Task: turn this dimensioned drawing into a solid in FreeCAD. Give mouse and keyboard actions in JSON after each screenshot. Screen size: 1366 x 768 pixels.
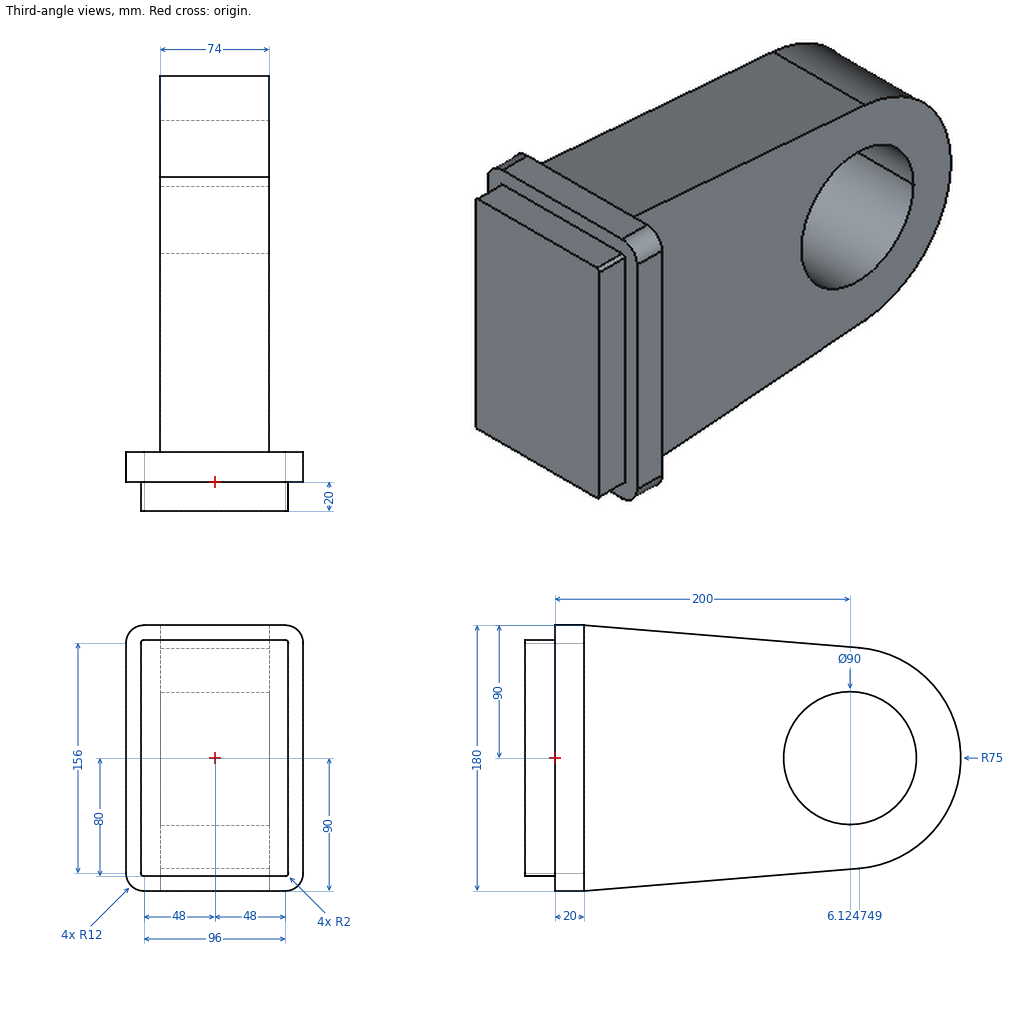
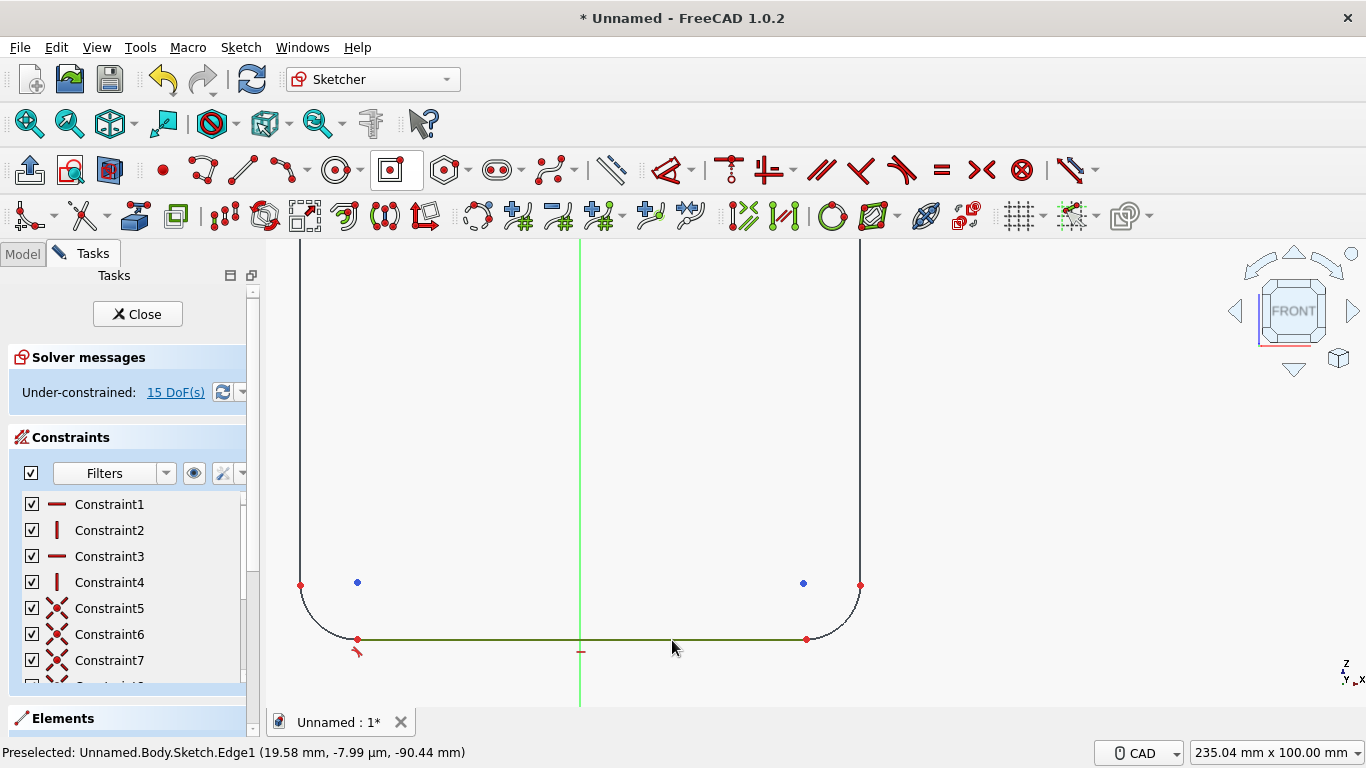
{"action": "left_click", "coordinate": [830, 633]}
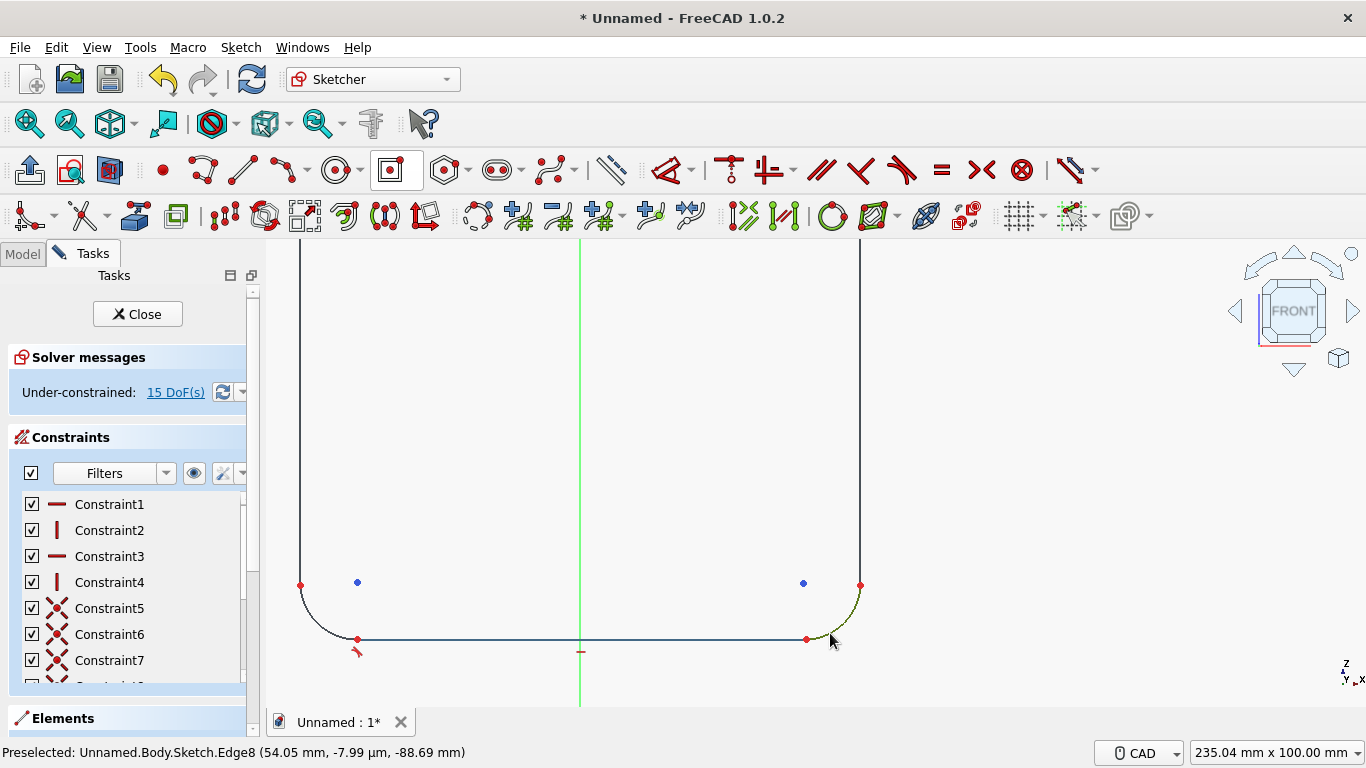
{"action": "left_click", "coordinate": [902, 170]}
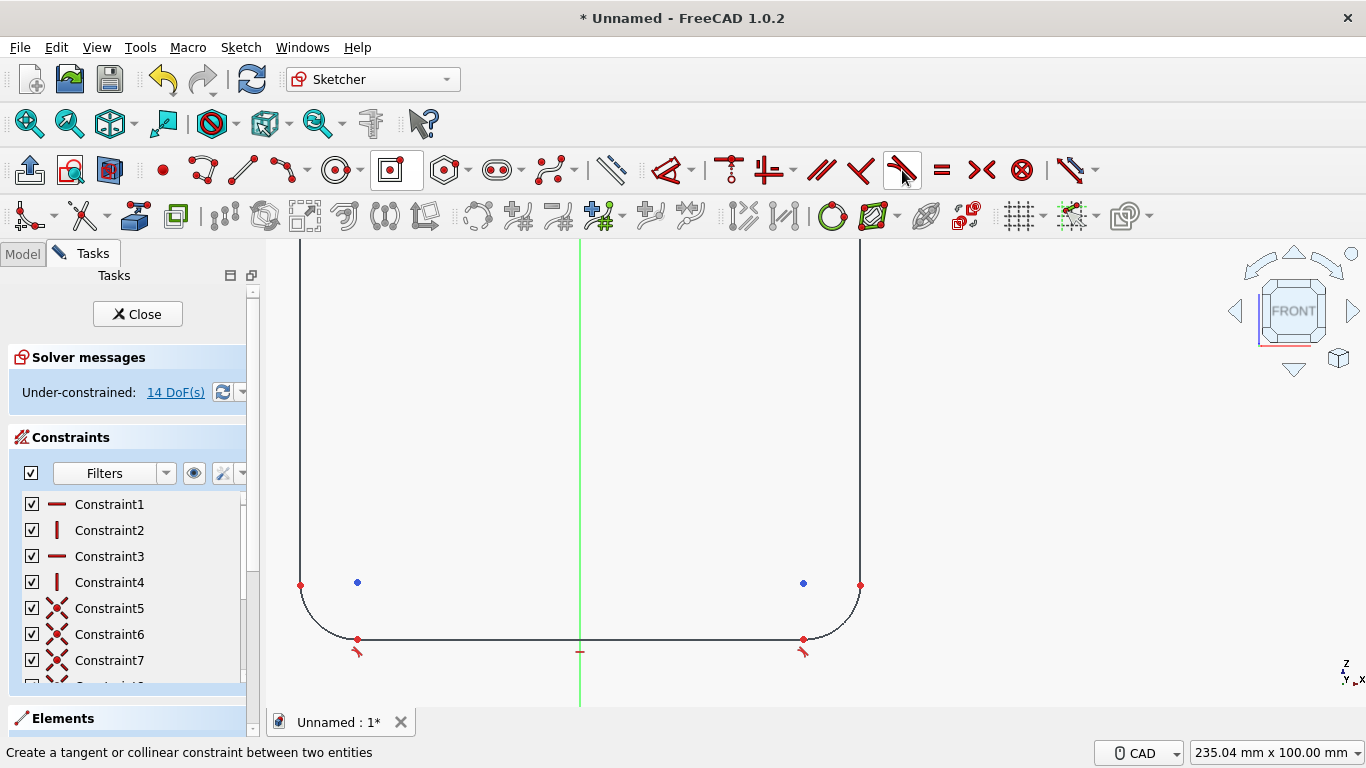
{"action": "left_click", "coordinate": [300, 366]}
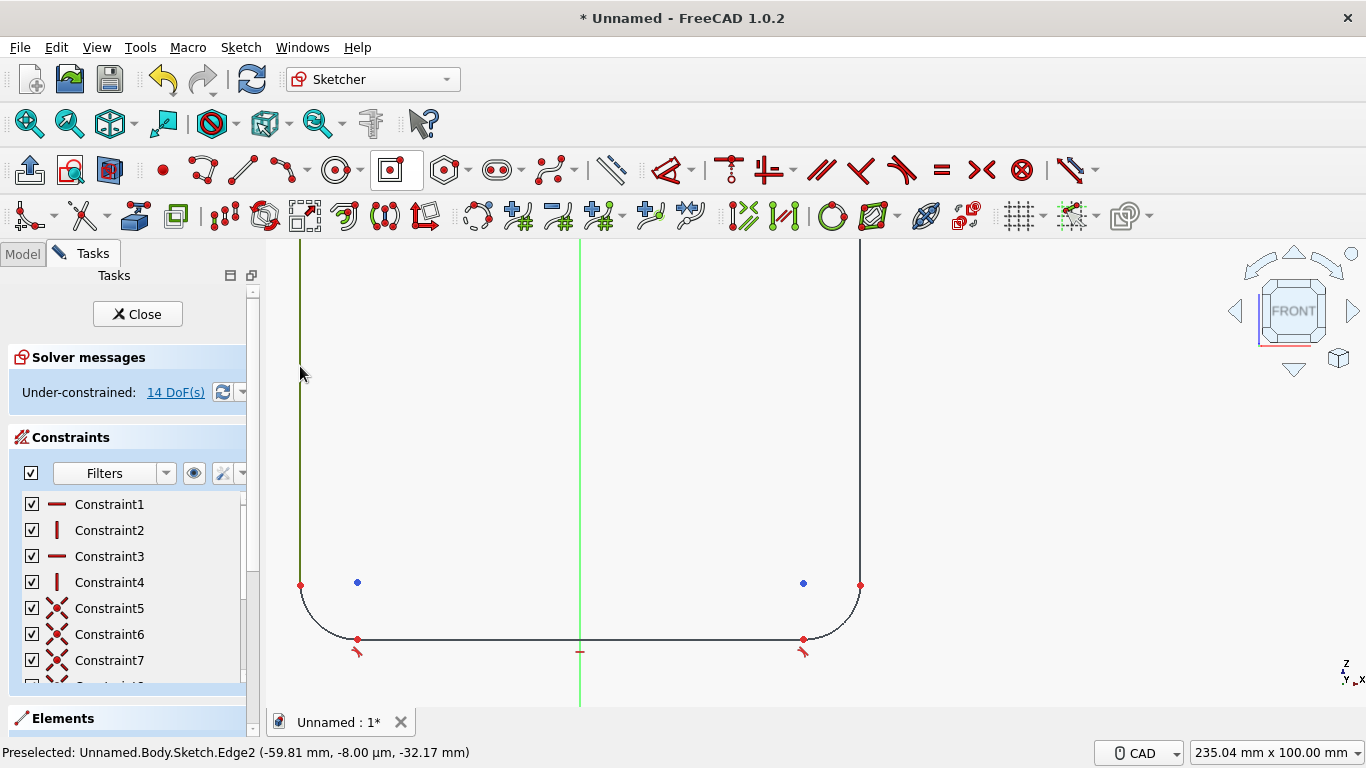
{"action": "left_click", "coordinate": [308, 610]}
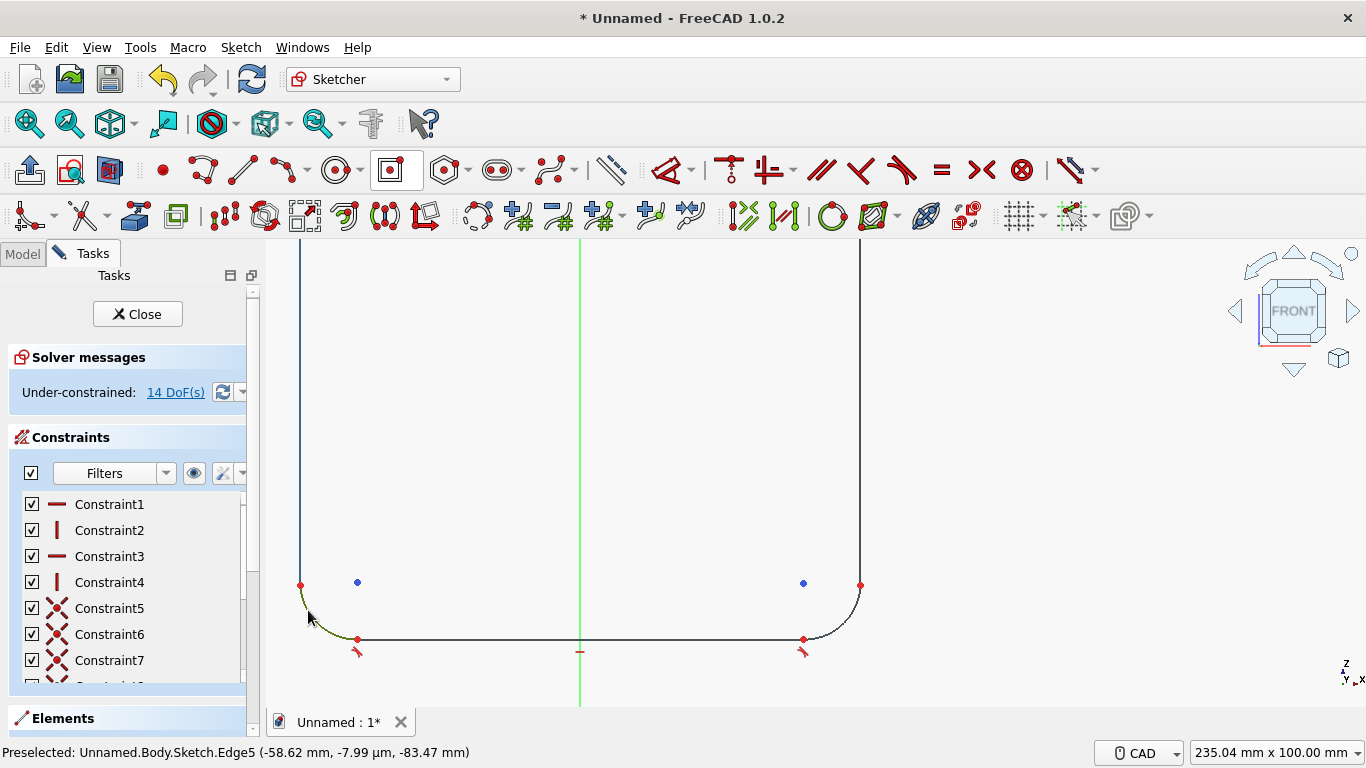
{"action": "key", "text": "t"}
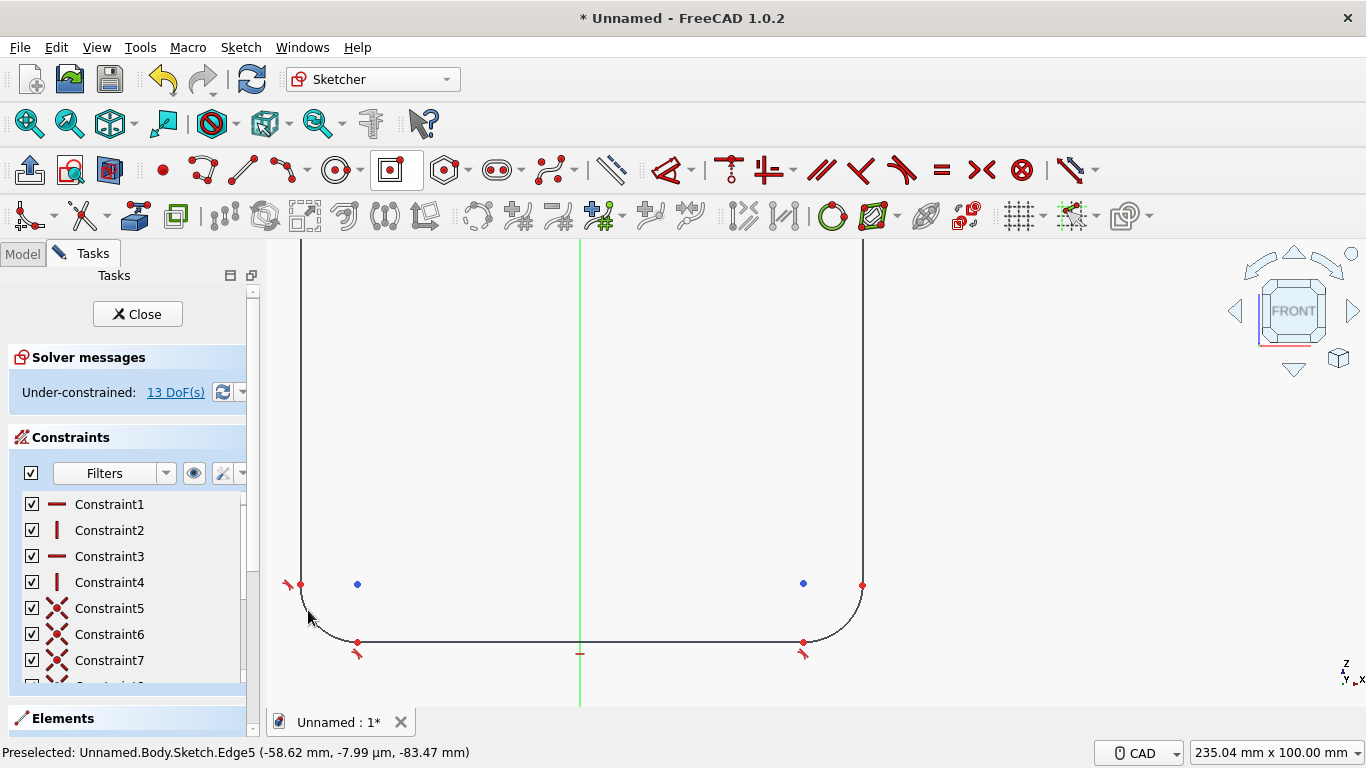
{"action": "left_click", "coordinate": [301, 366]}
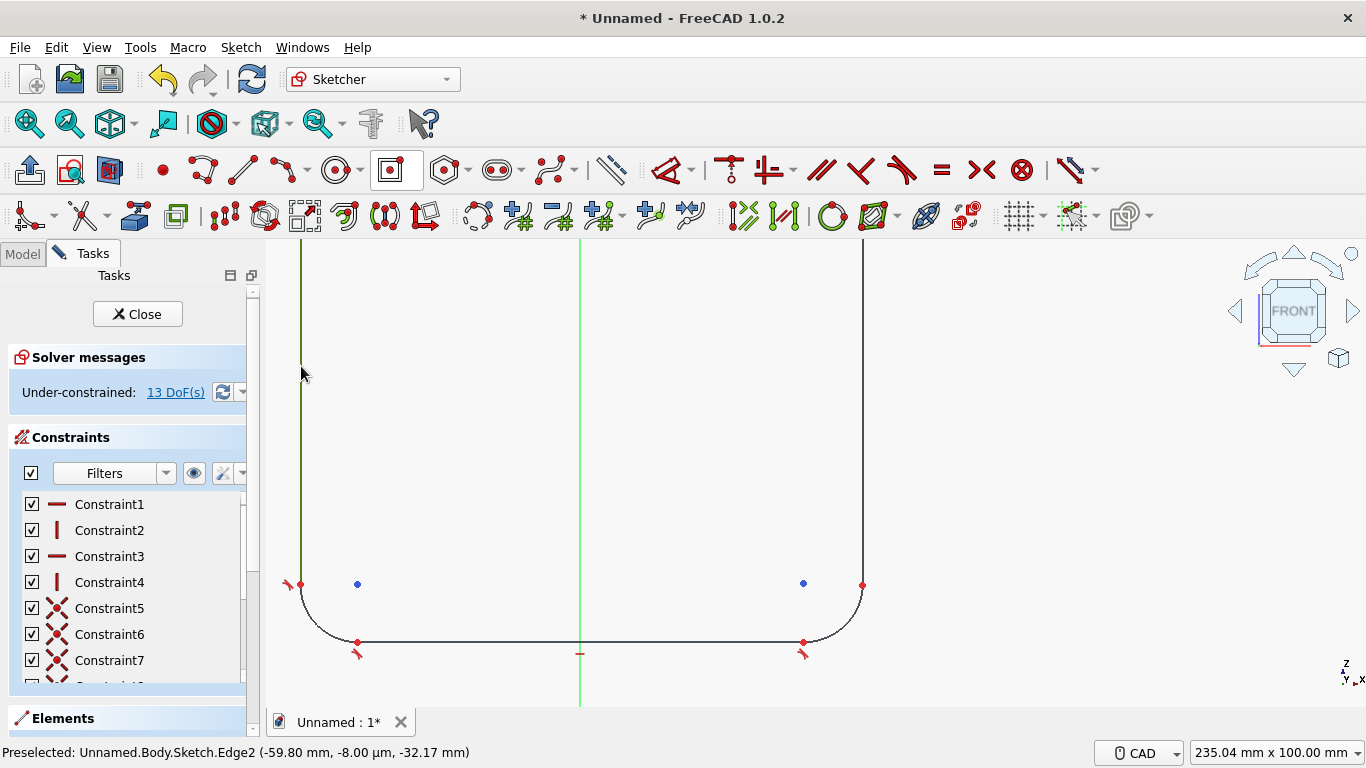
{"action": "scroll", "coordinate": [845, 622], "scroll_direction": "down", "scroll_amount": 5}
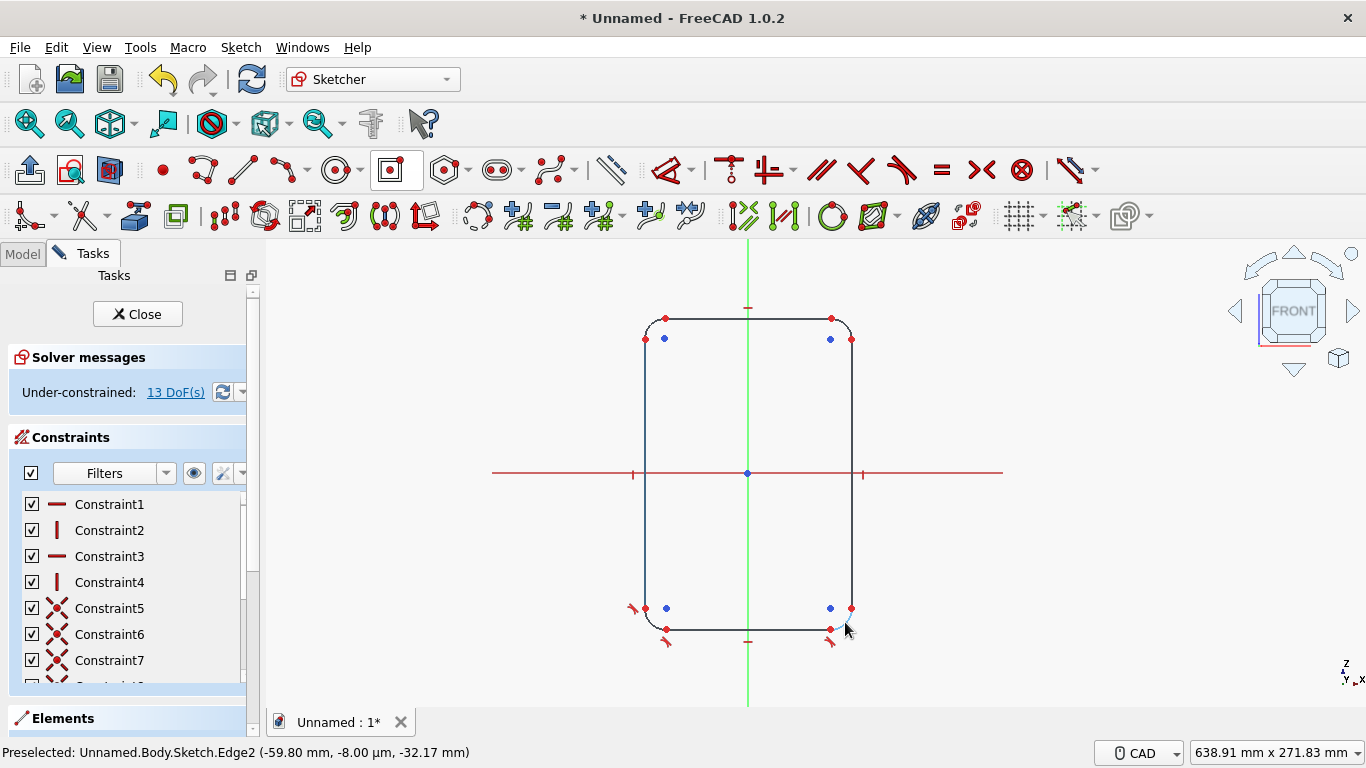
{"action": "scroll", "coordinate": [656, 321], "scroll_direction": "up", "scroll_amount": 2}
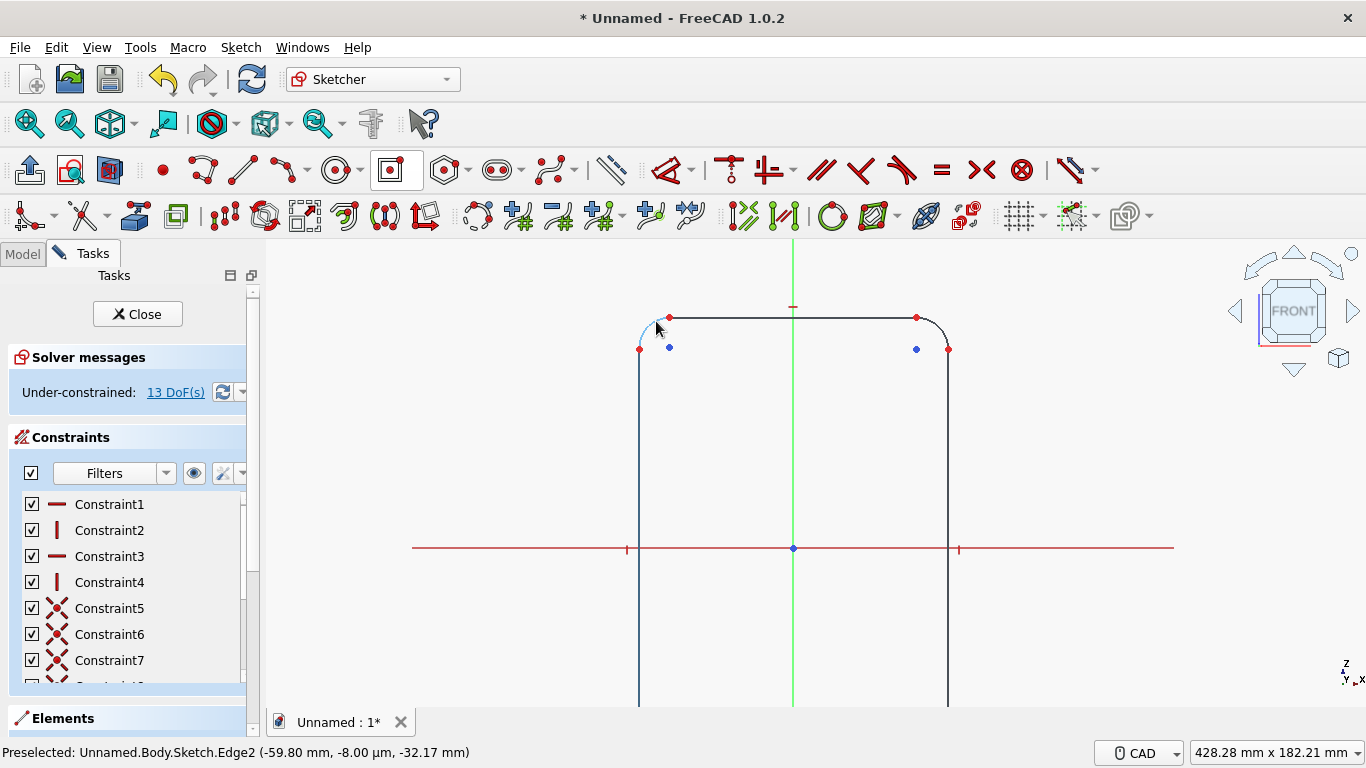
{"action": "left_click", "coordinate": [655, 321]}